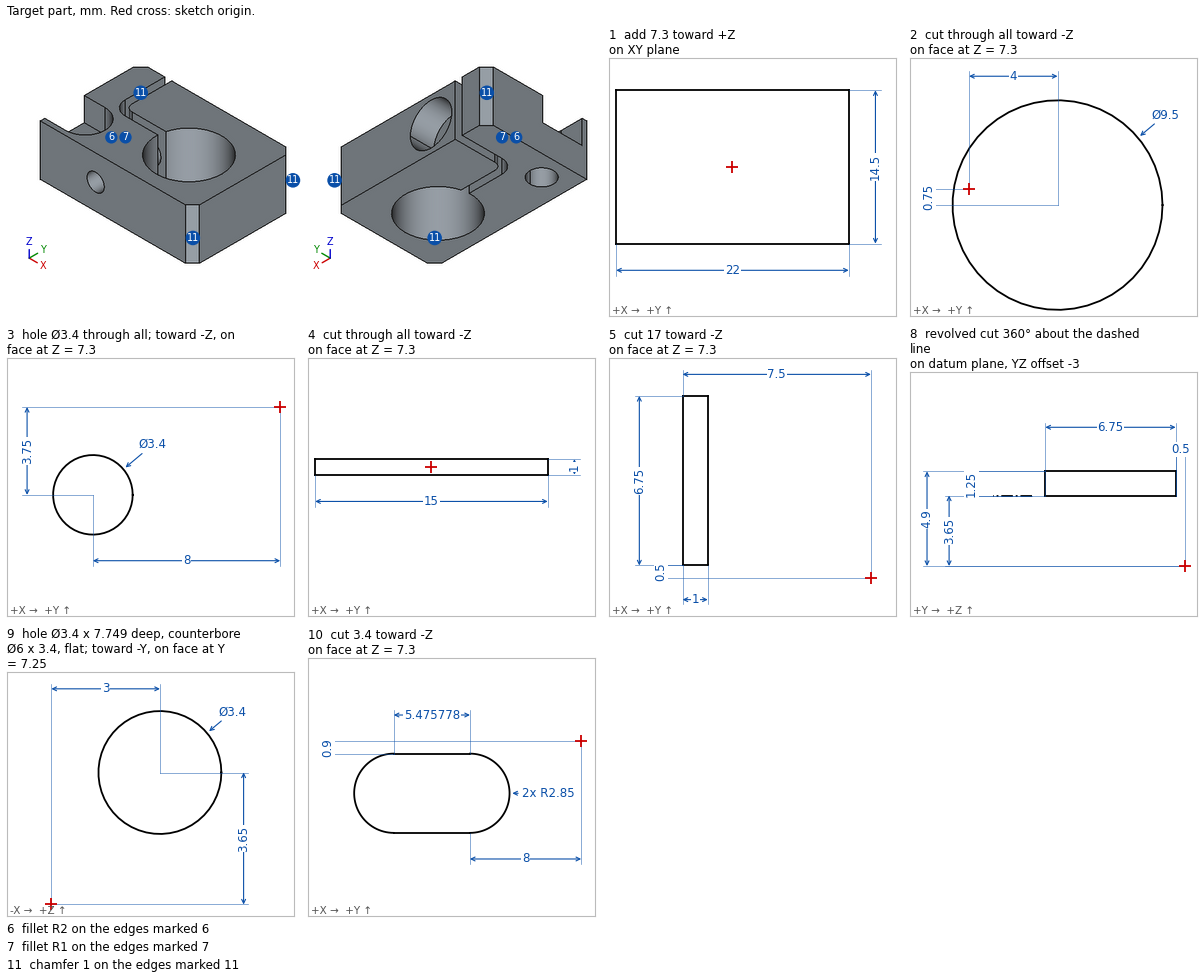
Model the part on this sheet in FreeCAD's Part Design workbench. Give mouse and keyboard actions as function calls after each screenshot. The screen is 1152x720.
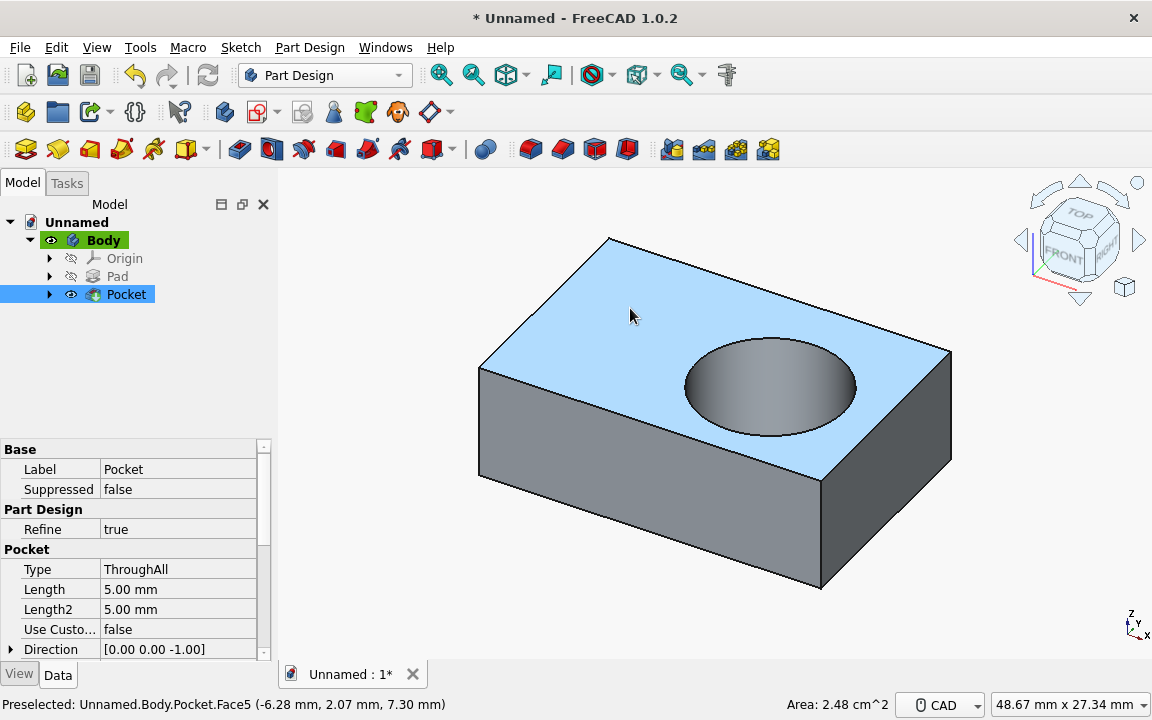
click(258, 112)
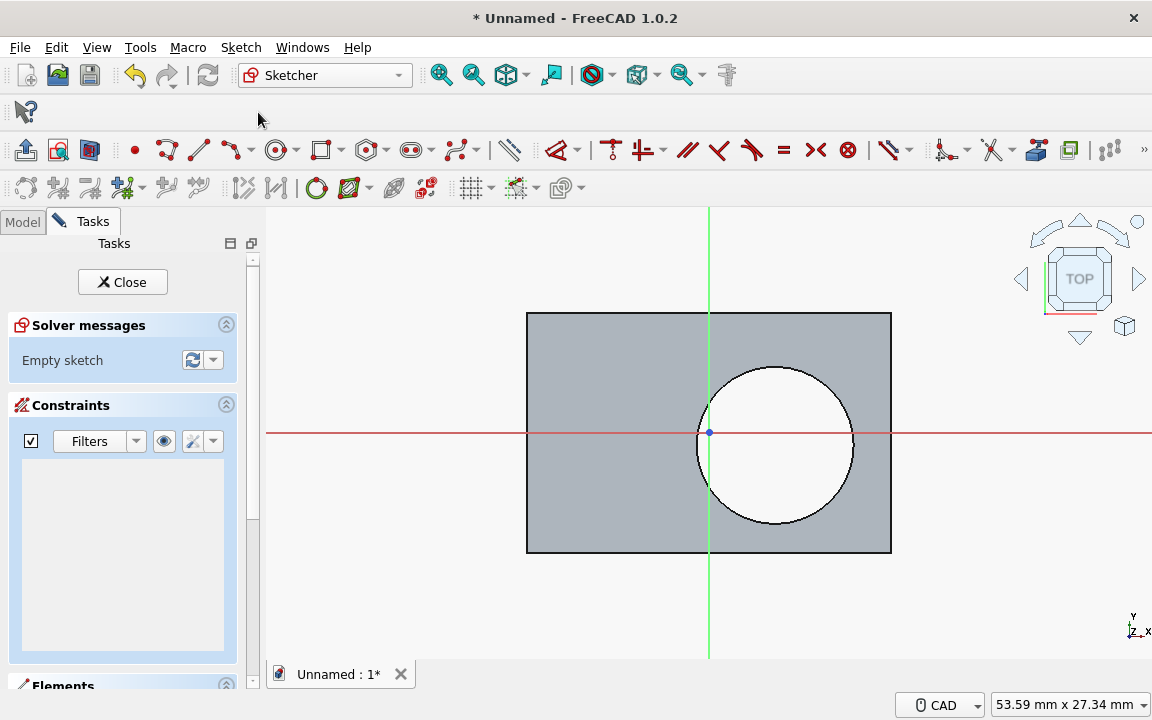
scroll(561, 511, up, 8)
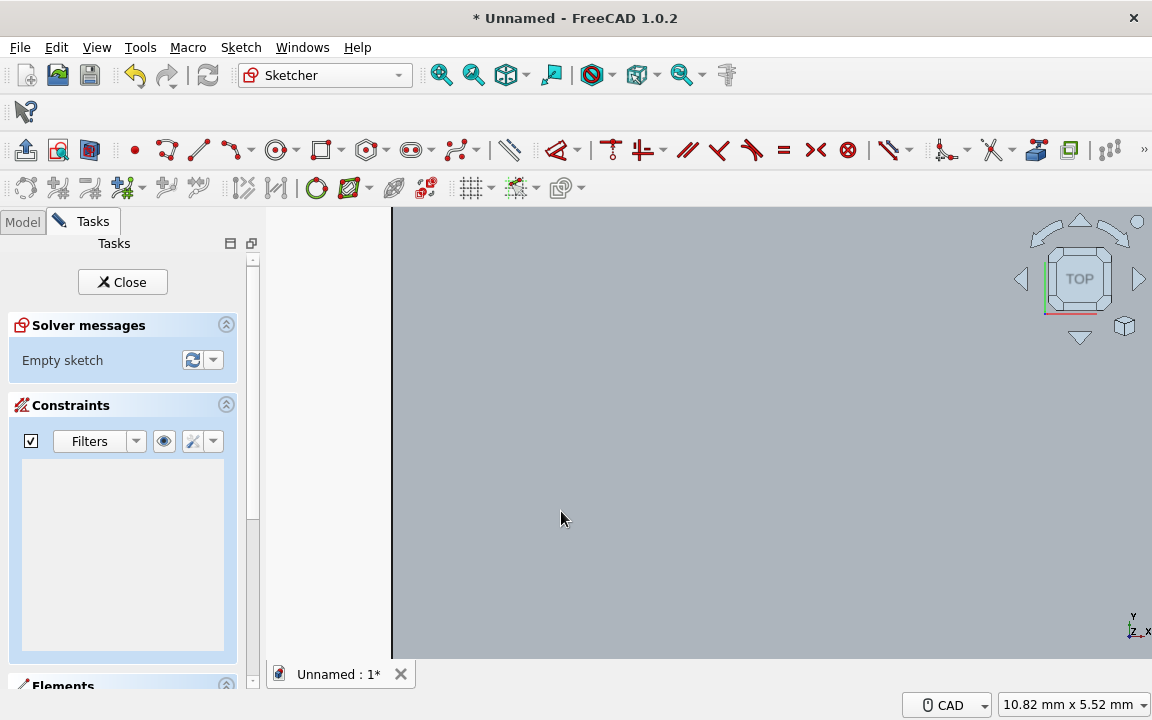
key(g)
key(c)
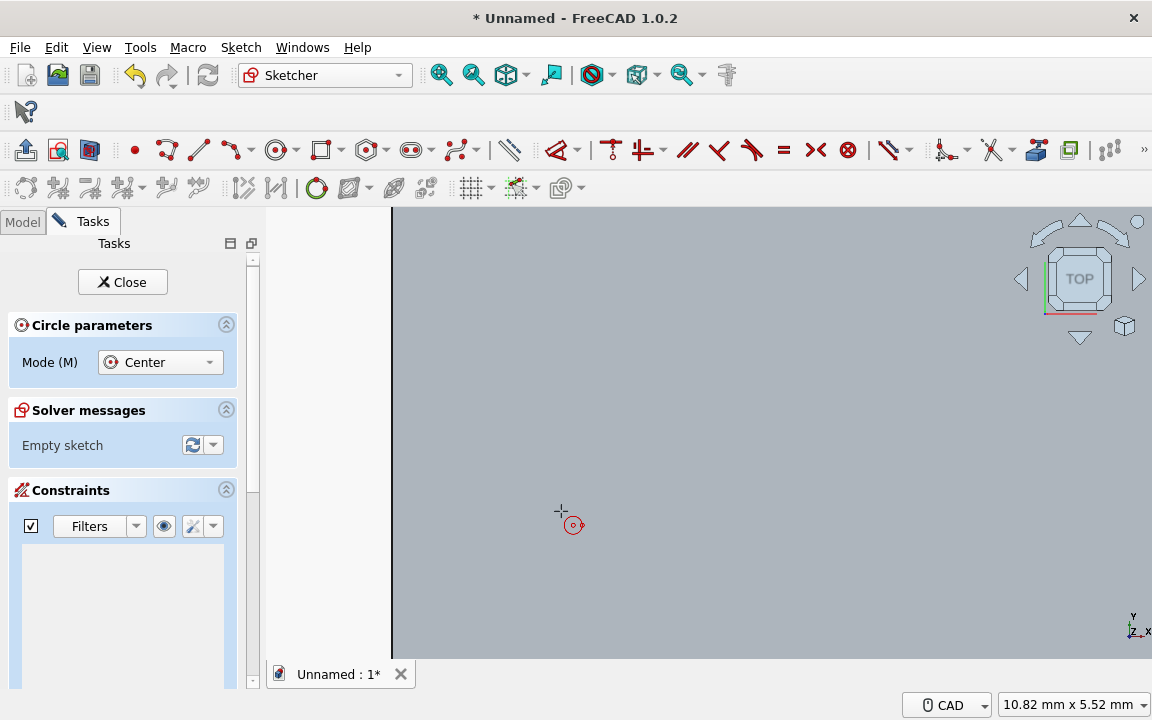
click(638, 429)
click(736, 331)
key(Escape)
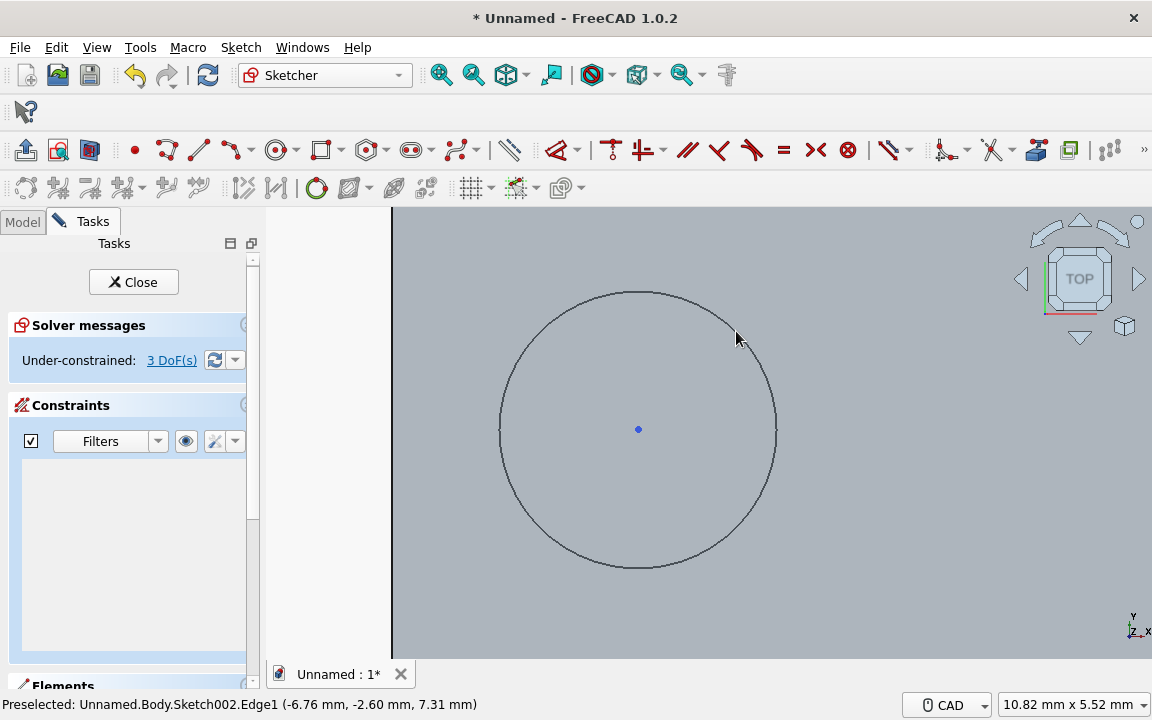
click(556, 150)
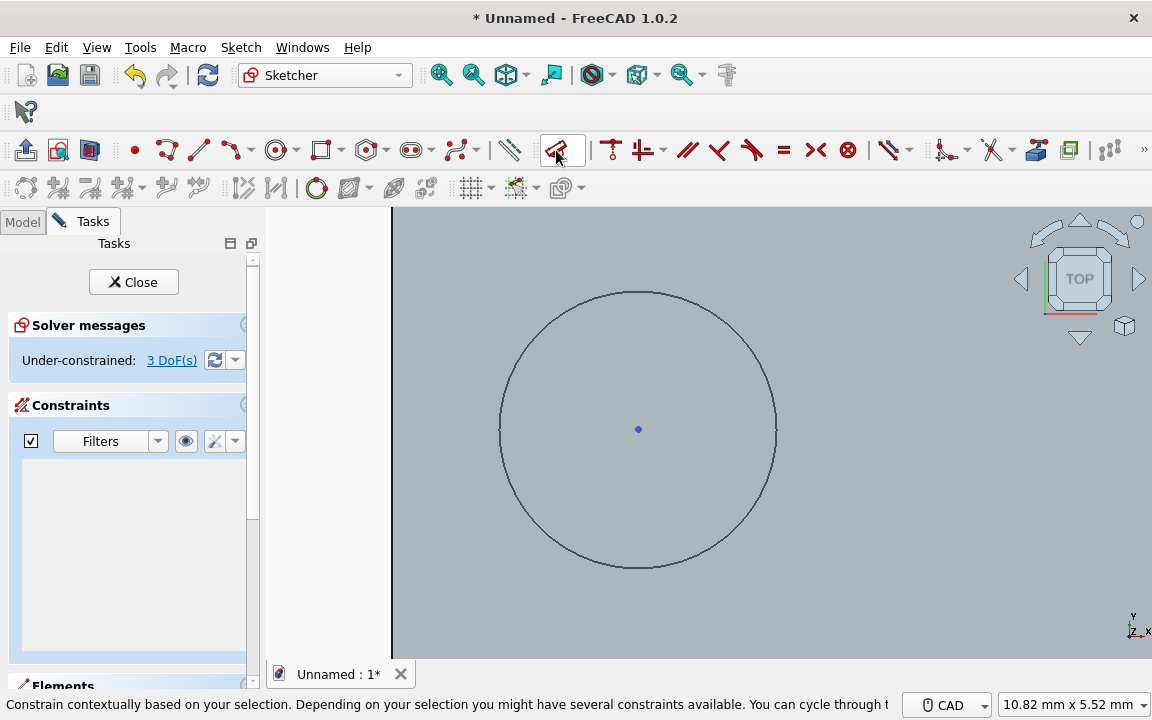
click(736, 332)
click(759, 309)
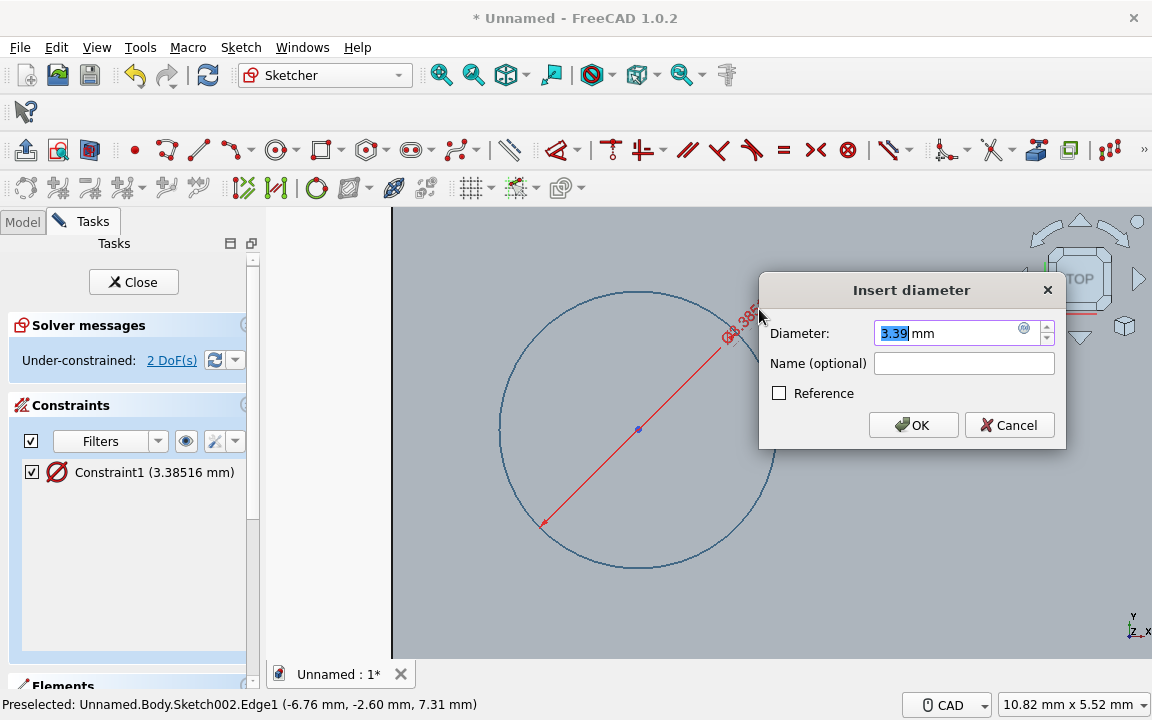
text(3.4)
key(Return)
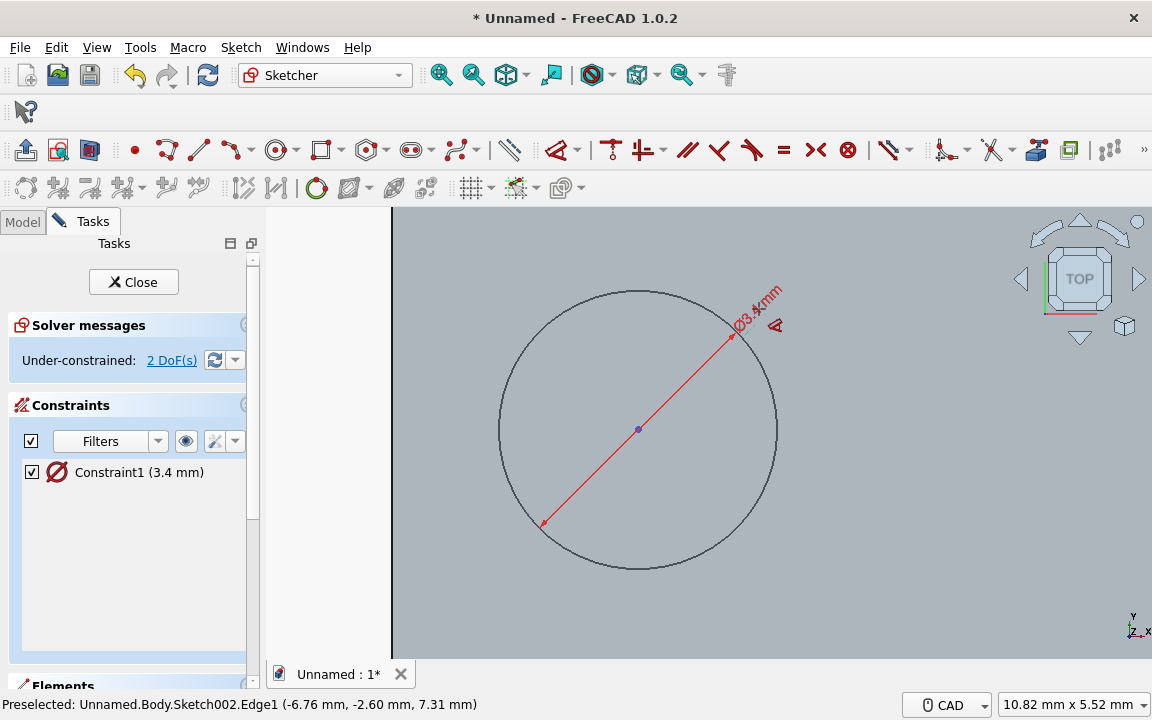
click(638, 430)
click(812, 464)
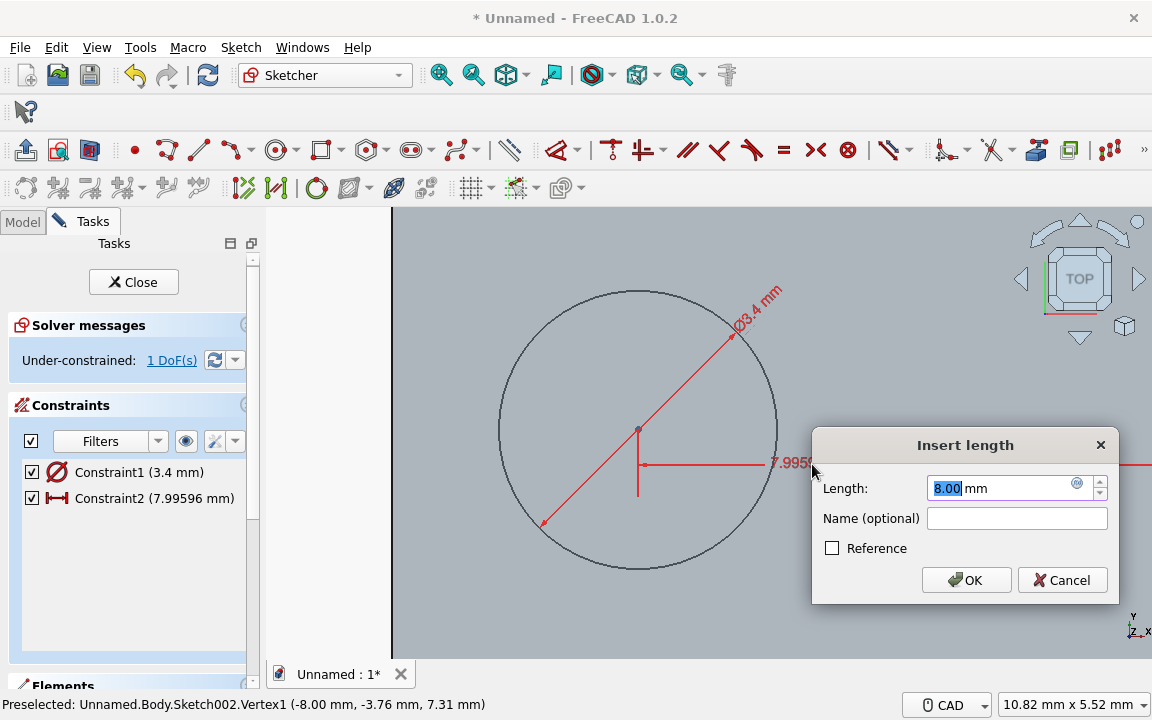
text(8)
key(Return)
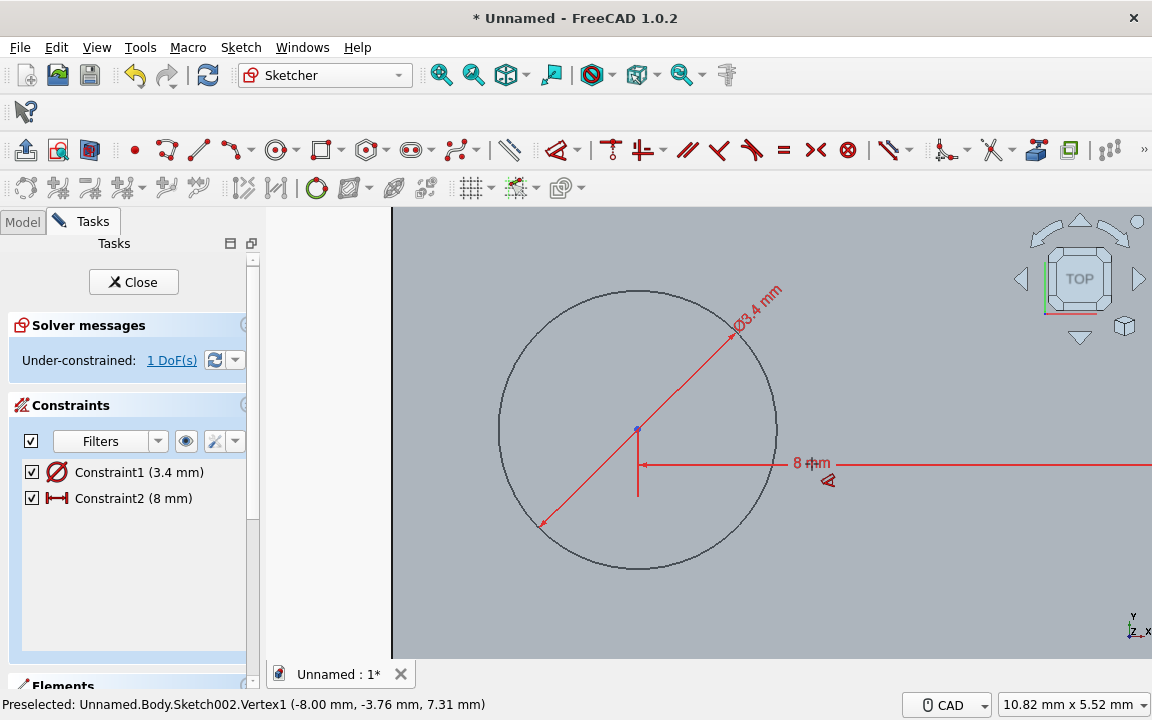
click(638, 430)
click(604, 332)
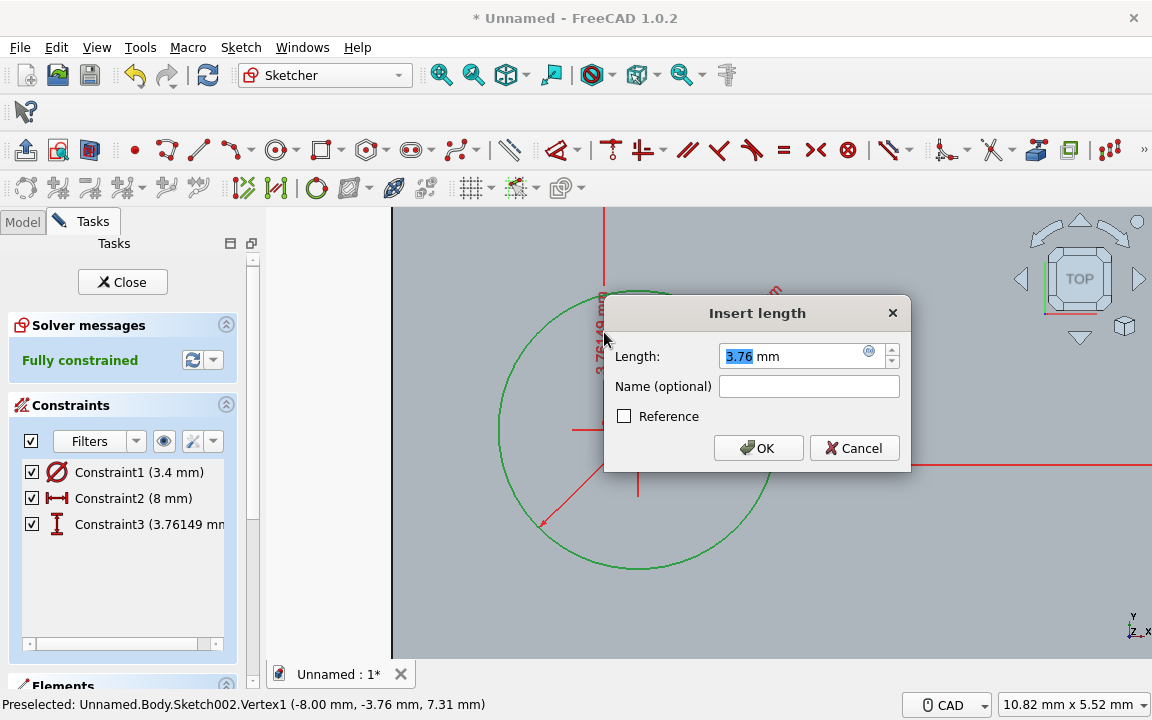
text(3.75)
key(Return)
key(Escape)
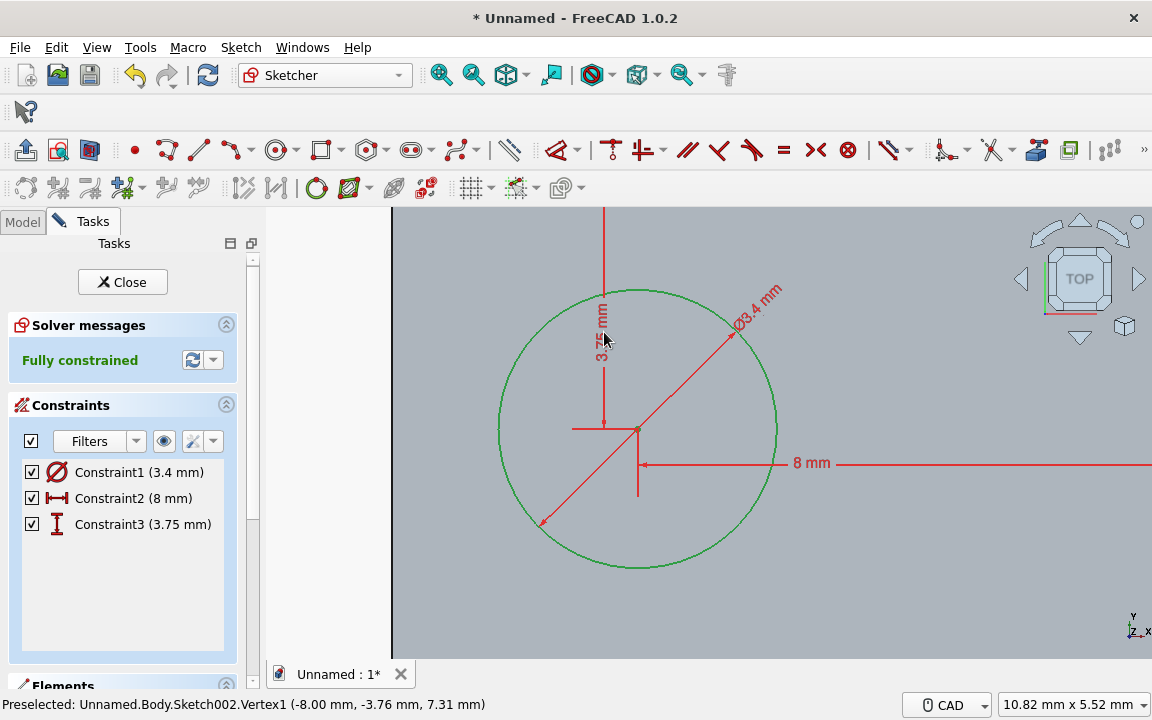
click(123, 282)